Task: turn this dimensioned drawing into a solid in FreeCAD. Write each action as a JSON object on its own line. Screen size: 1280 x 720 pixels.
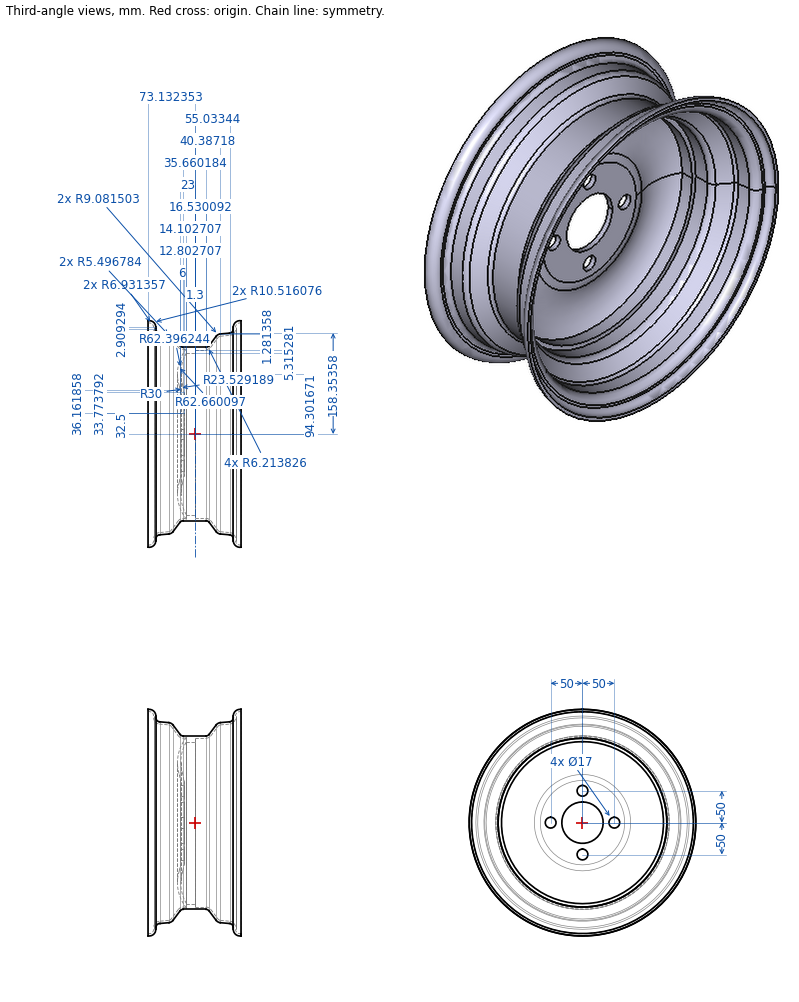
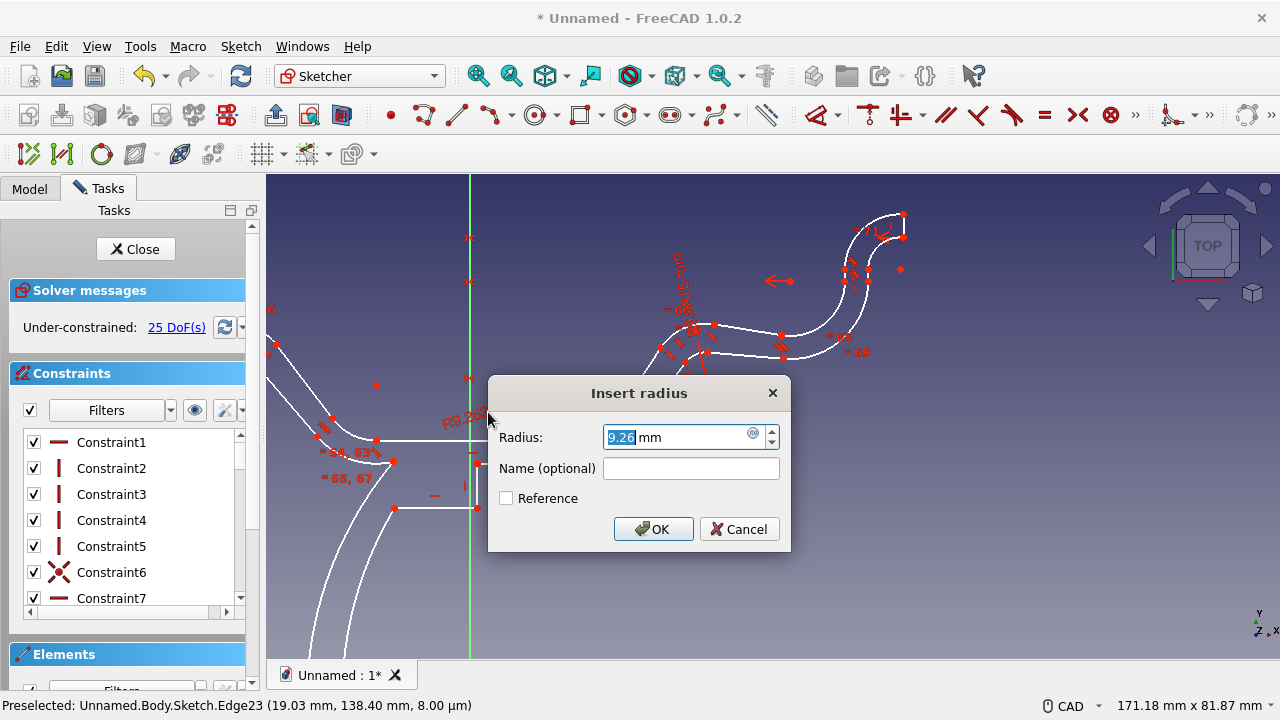
{"action": "type", "text": "6.213826"}
{"action": "key", "text": "Return"}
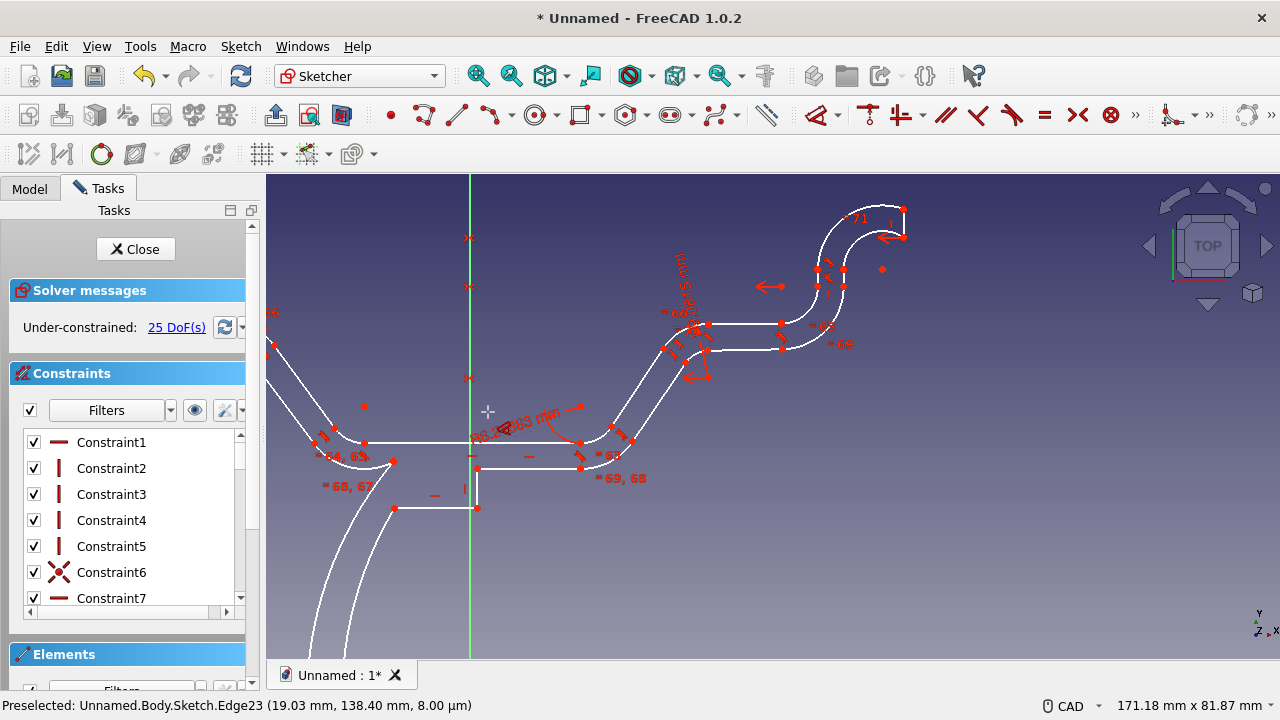
{"action": "scroll", "coordinate": [806, 280], "scroll_direction": "down", "scroll_amount": 6}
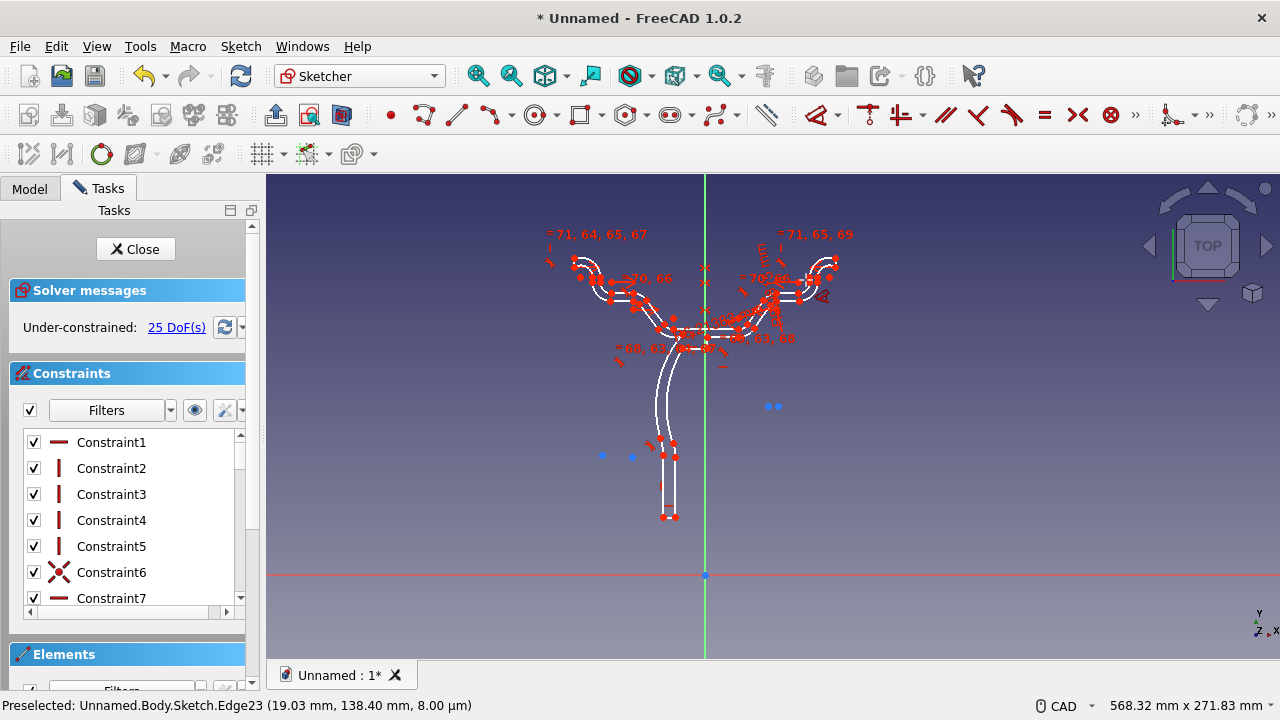
{"action": "scroll", "coordinate": [597, 267], "scroll_direction": "up", "scroll_amount": 4}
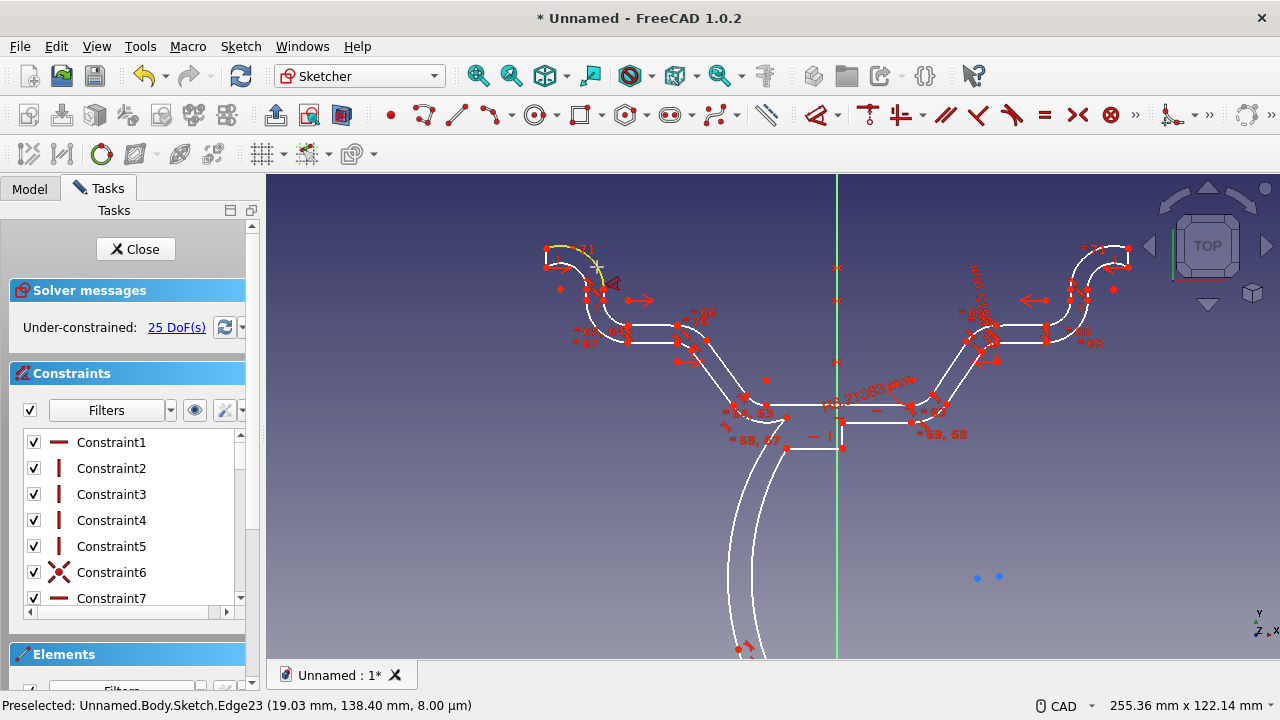
{"action": "left_click", "coordinate": [597, 266]}
{"action": "left_click", "coordinate": [624, 249]}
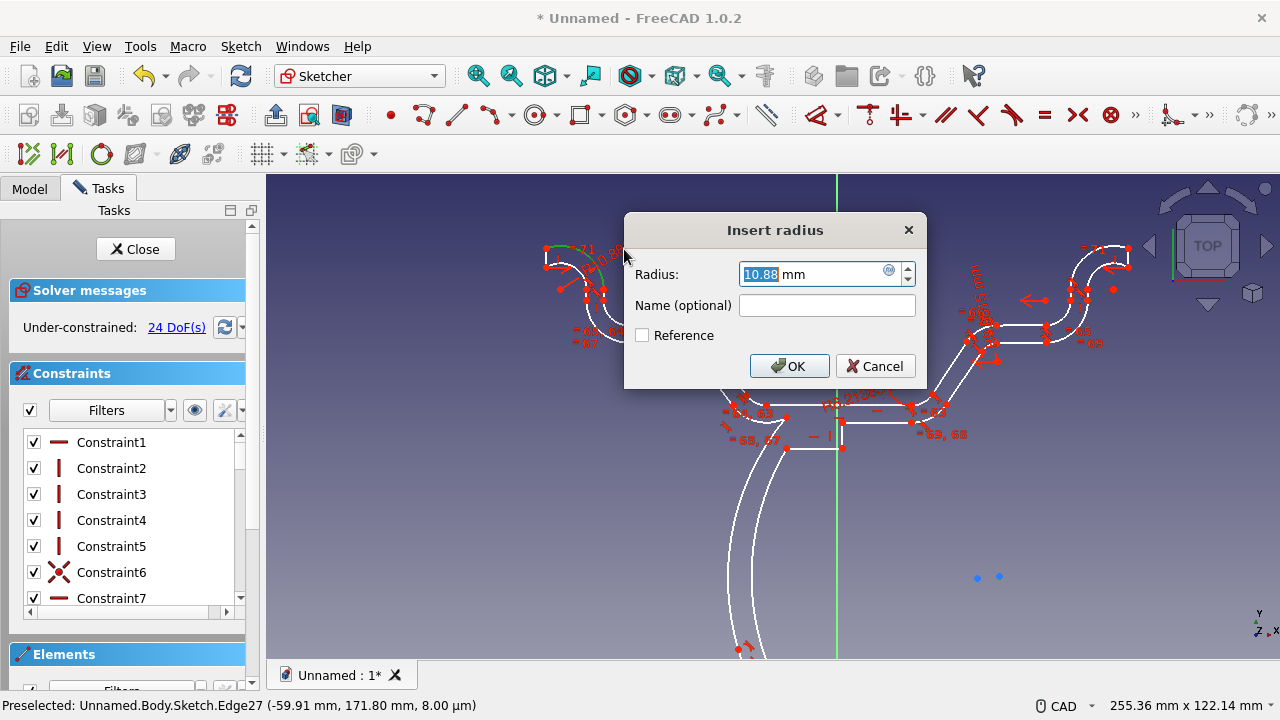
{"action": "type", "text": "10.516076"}
{"action": "key", "text": "Return"}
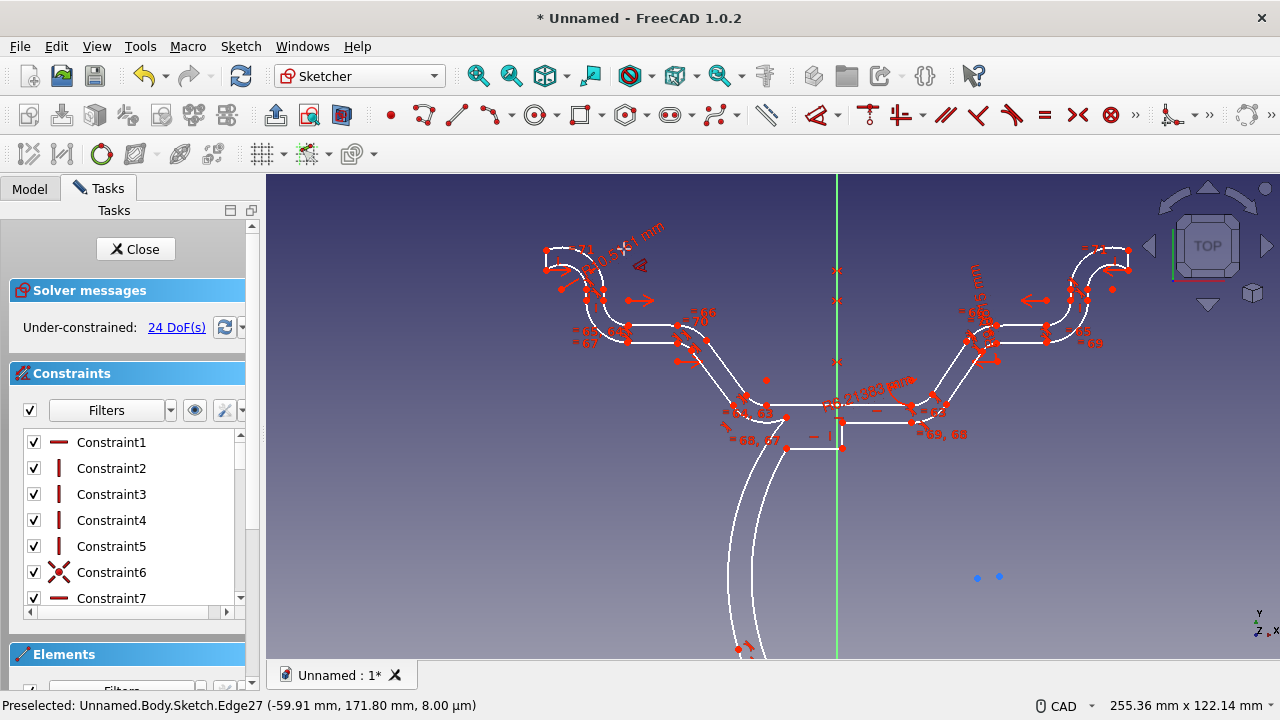
{"action": "scroll", "coordinate": [581, 274], "scroll_direction": "up", "scroll_amount": 2}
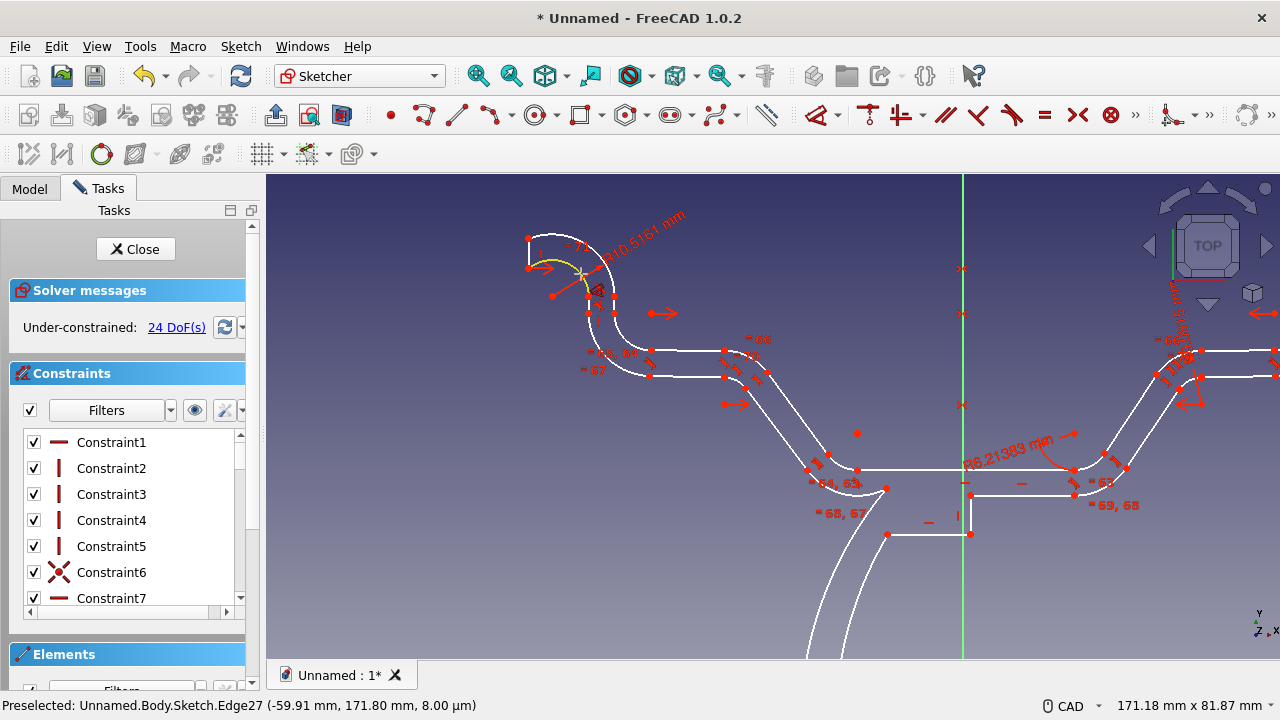
{"action": "left_click", "coordinate": [581, 274]}
{"action": "left_click", "coordinate": [510, 243]}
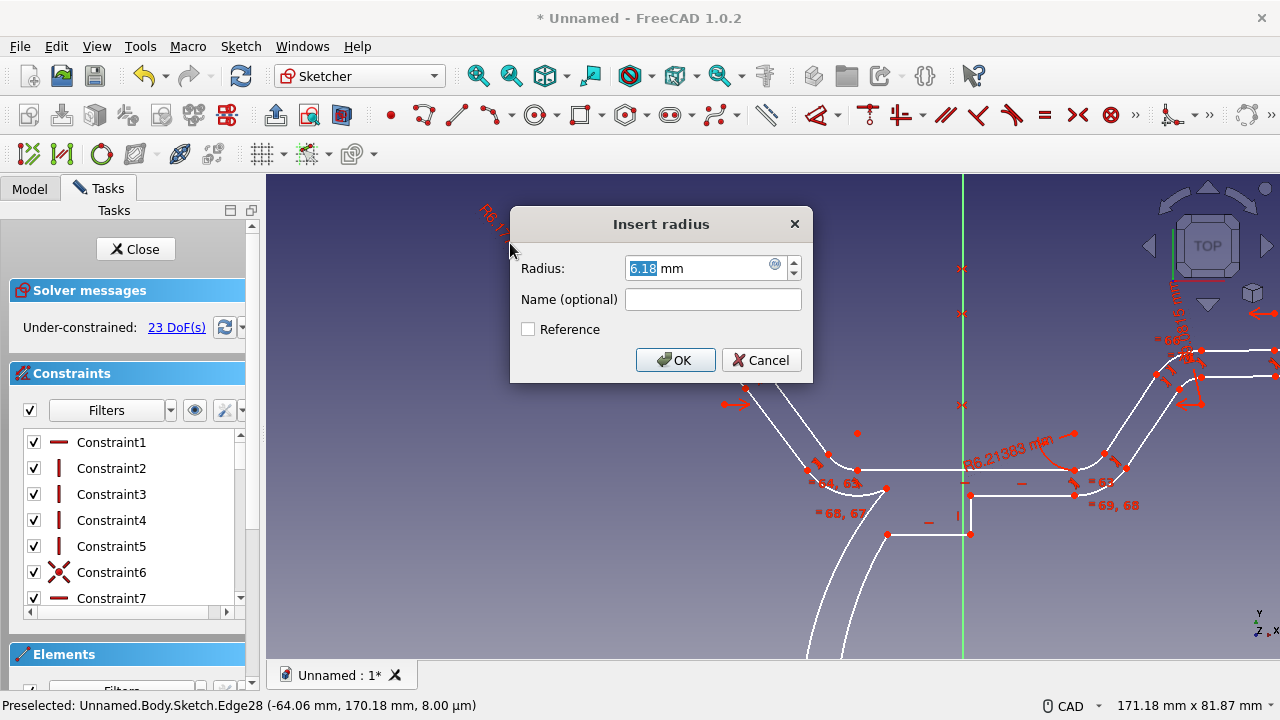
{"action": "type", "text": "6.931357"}
{"action": "key", "text": "Return"}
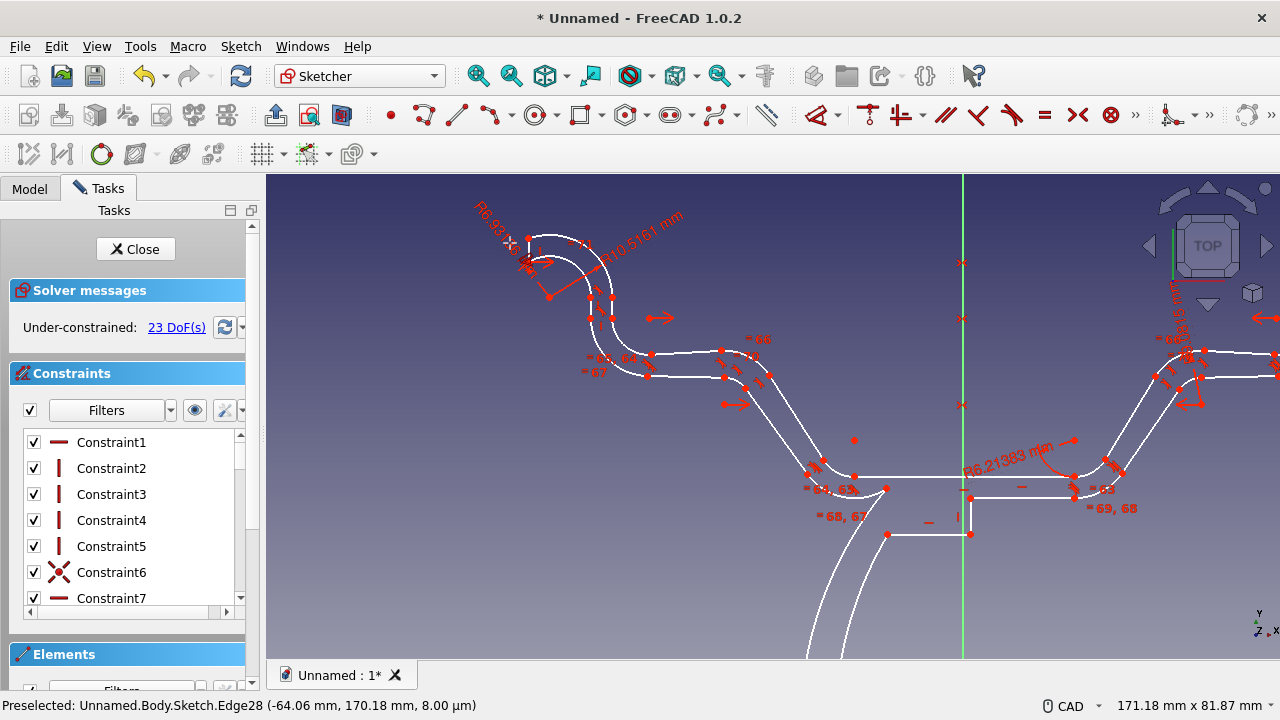
{"action": "left_click", "coordinate": [737, 381]}
{"action": "left_click", "coordinate": [696, 456]}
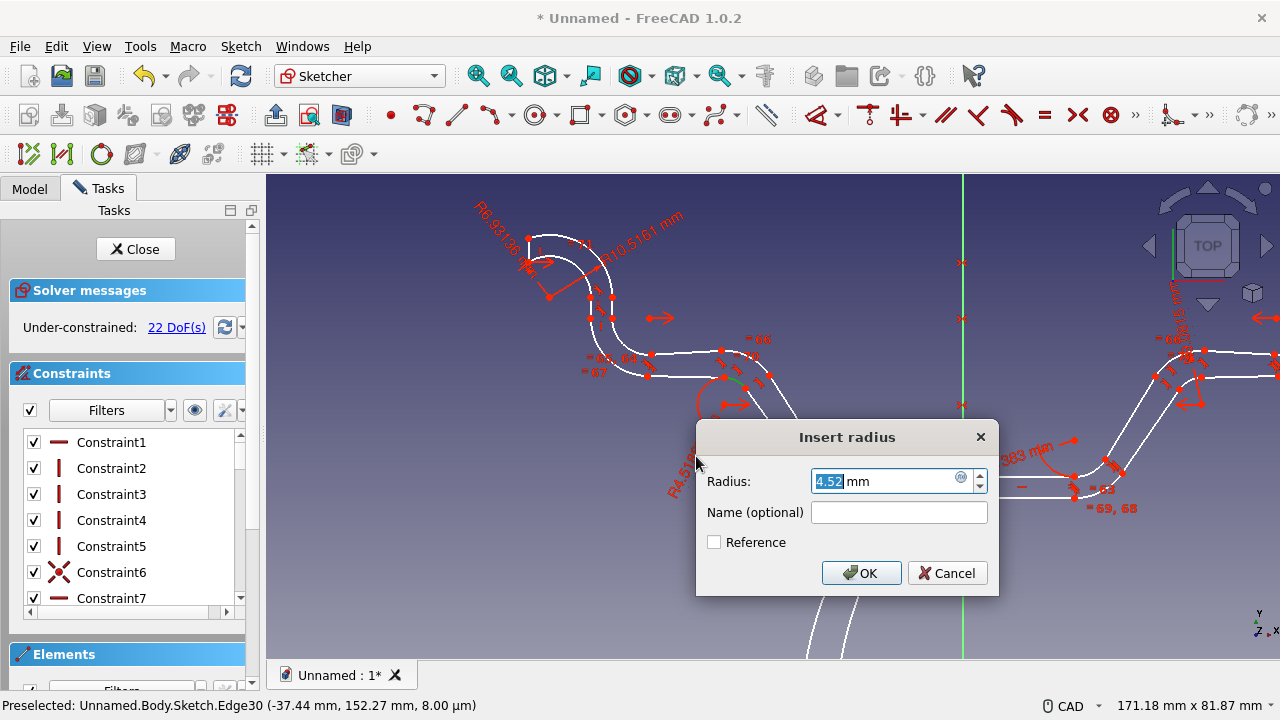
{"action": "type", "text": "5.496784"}
{"action": "key", "text": "Return"}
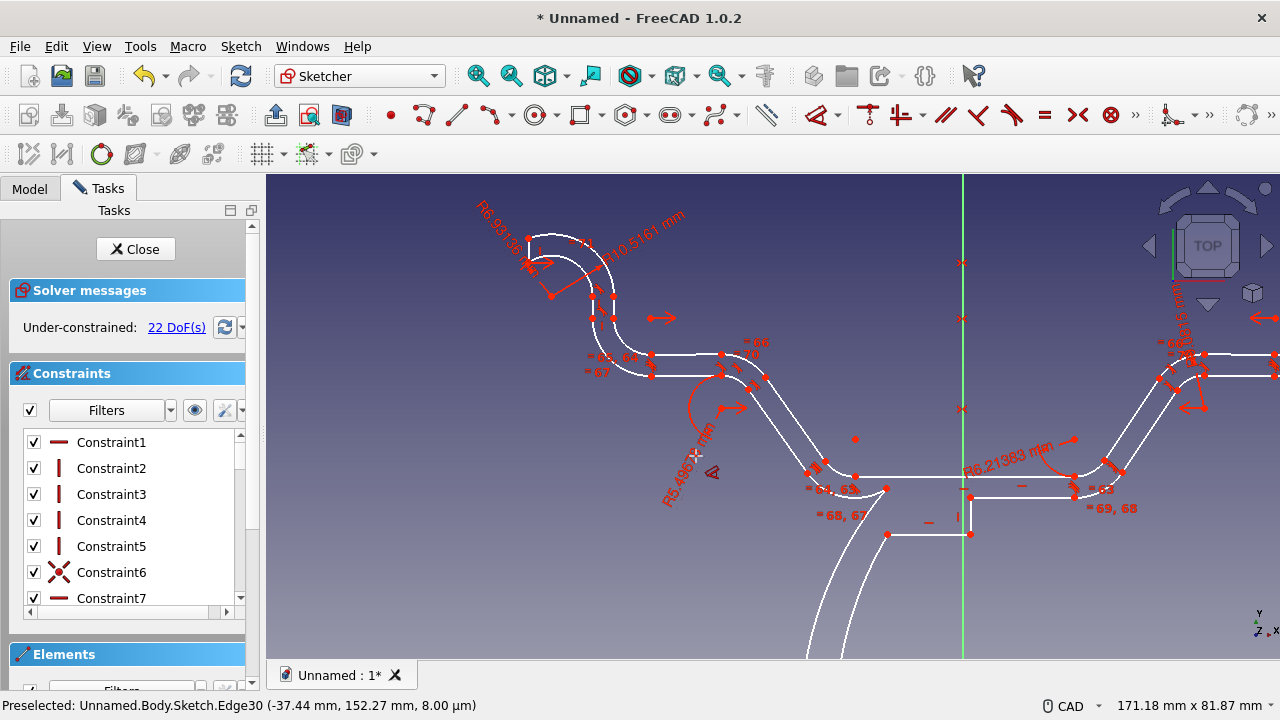
{"action": "left_click", "coordinate": [830, 582]}
{"action": "left_click", "coordinate": [801, 570]}